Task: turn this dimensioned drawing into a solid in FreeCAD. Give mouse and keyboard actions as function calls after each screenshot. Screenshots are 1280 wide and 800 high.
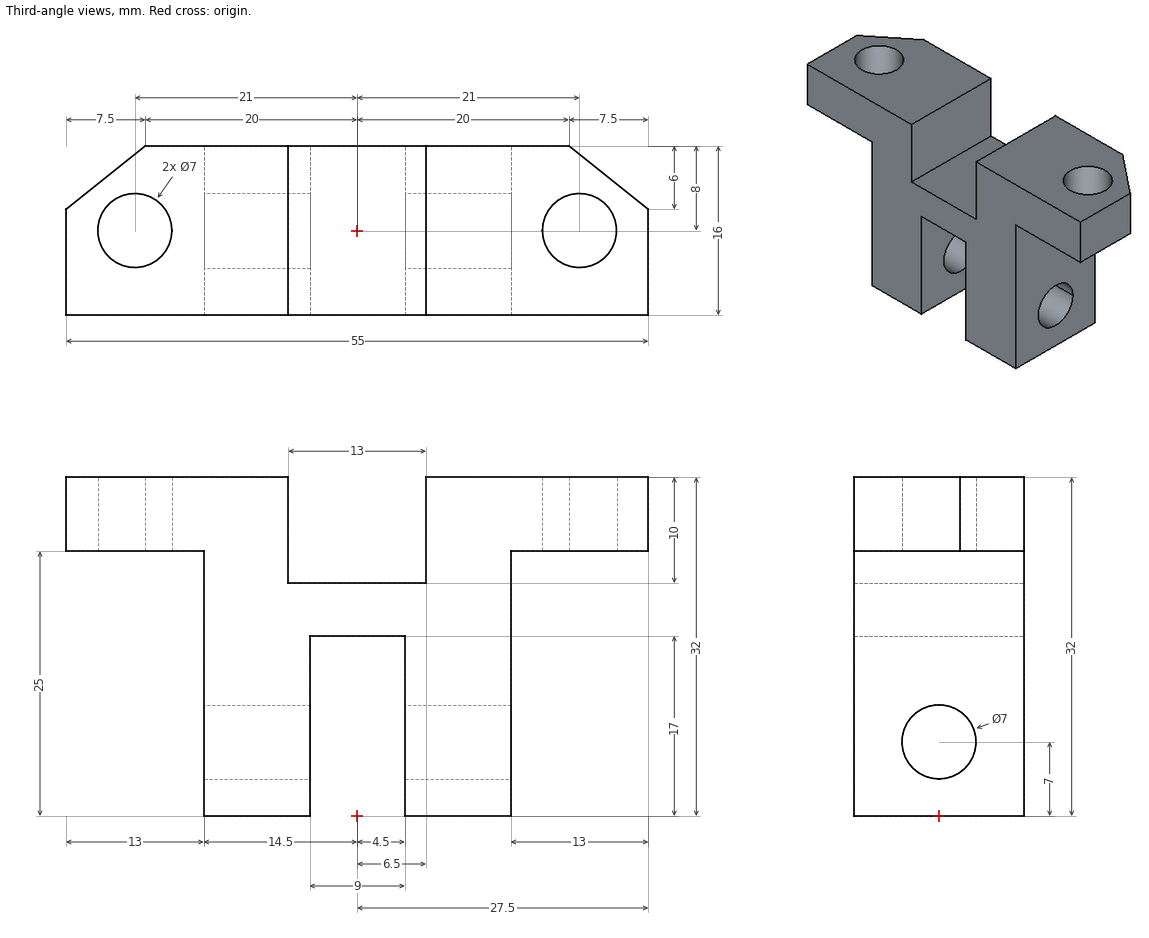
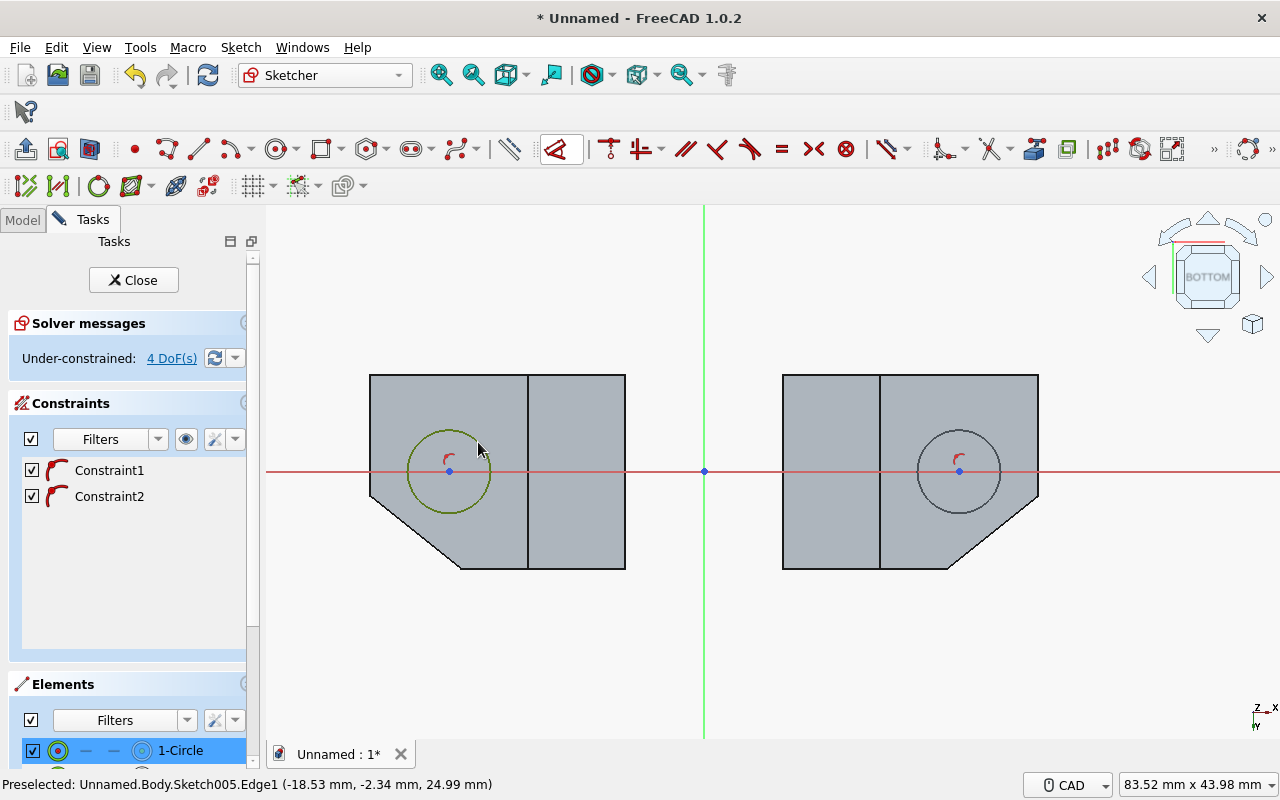
click(988, 442)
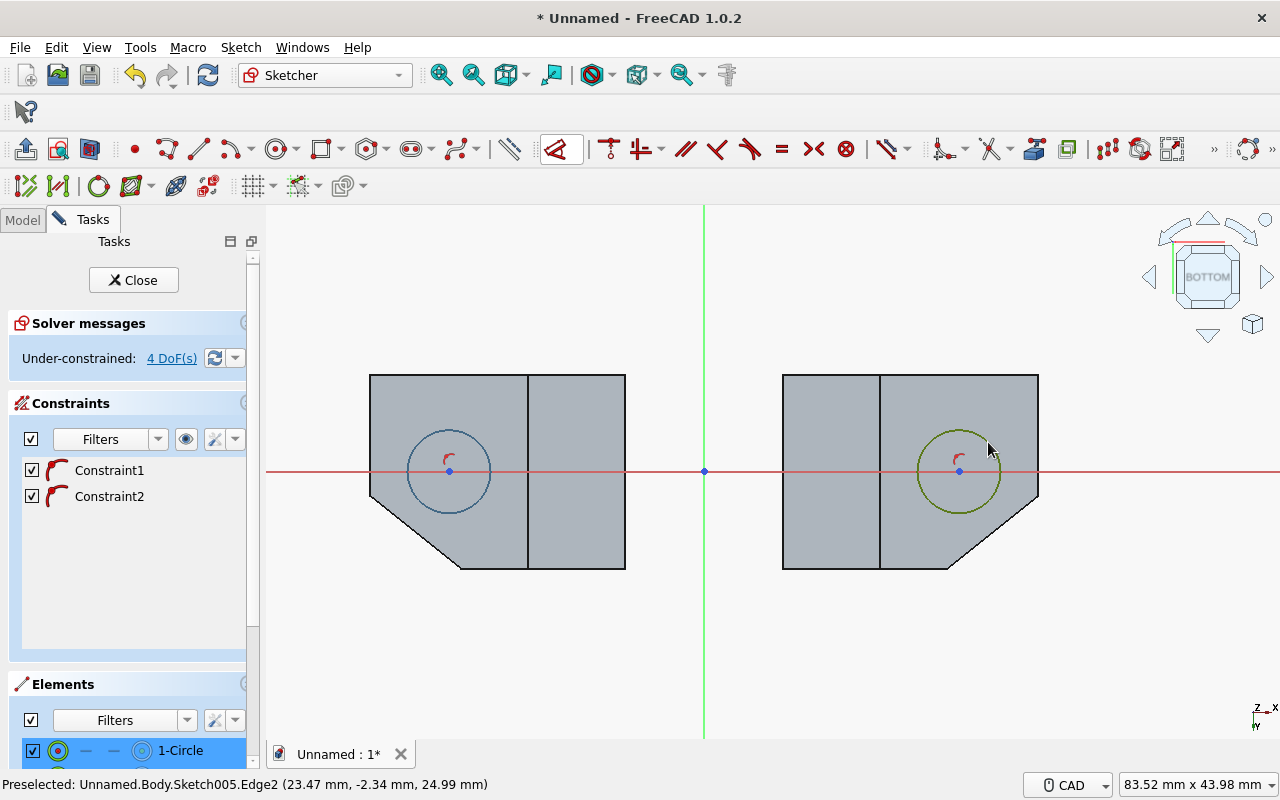
key(e)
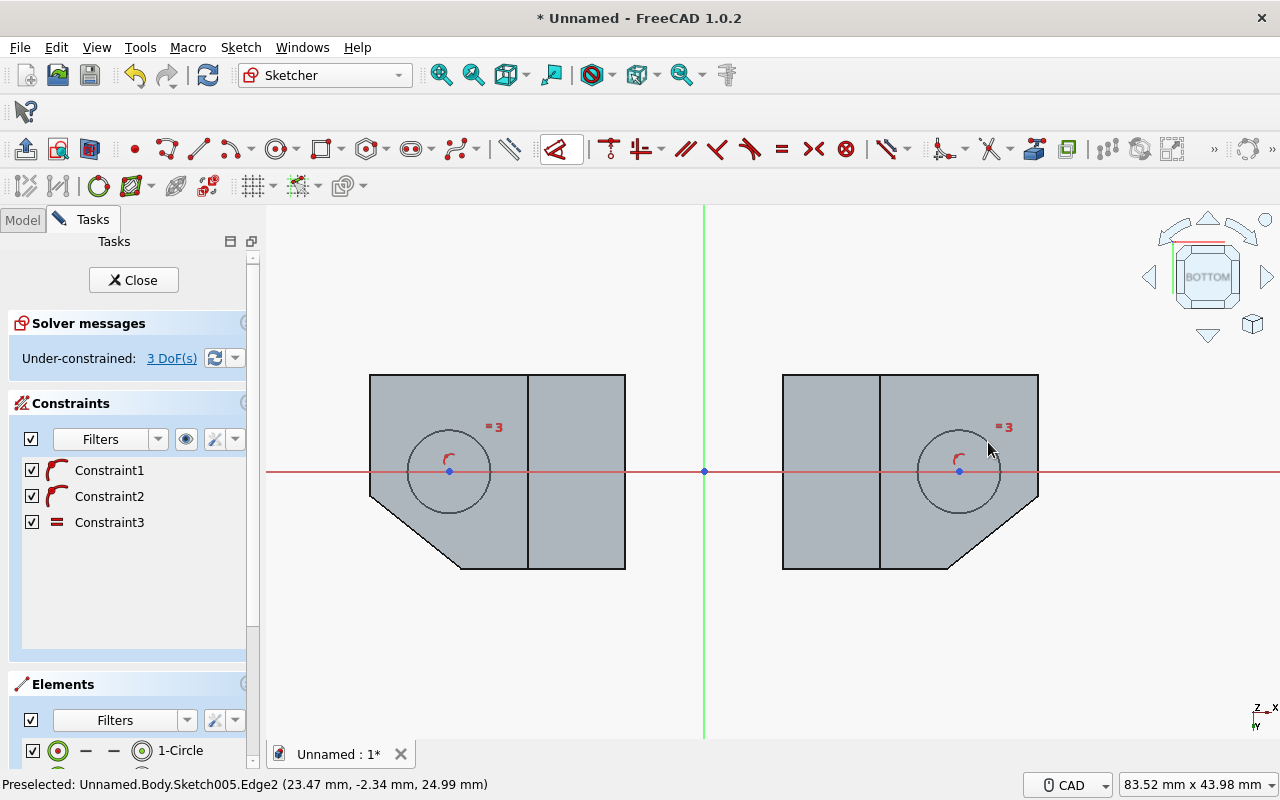
click(478, 442)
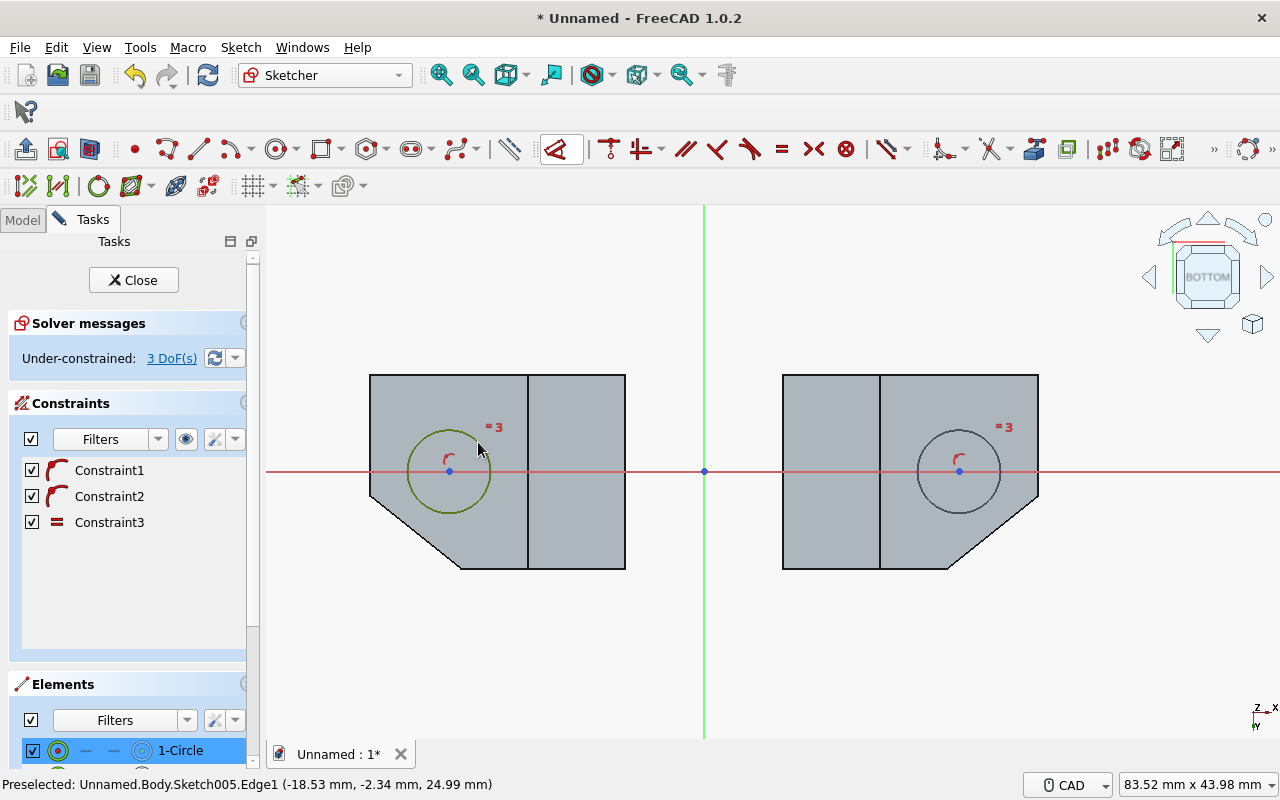
key(k)
key(o)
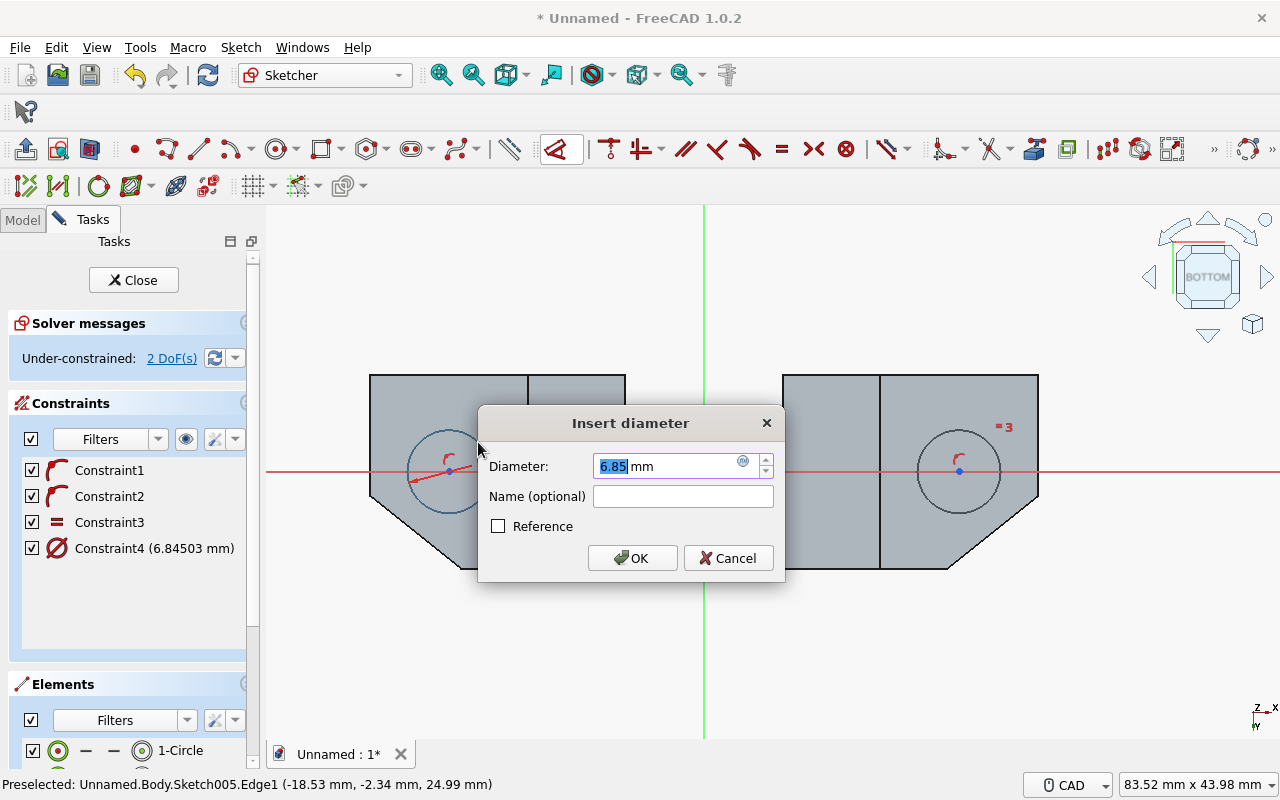
text(7)
key(Return)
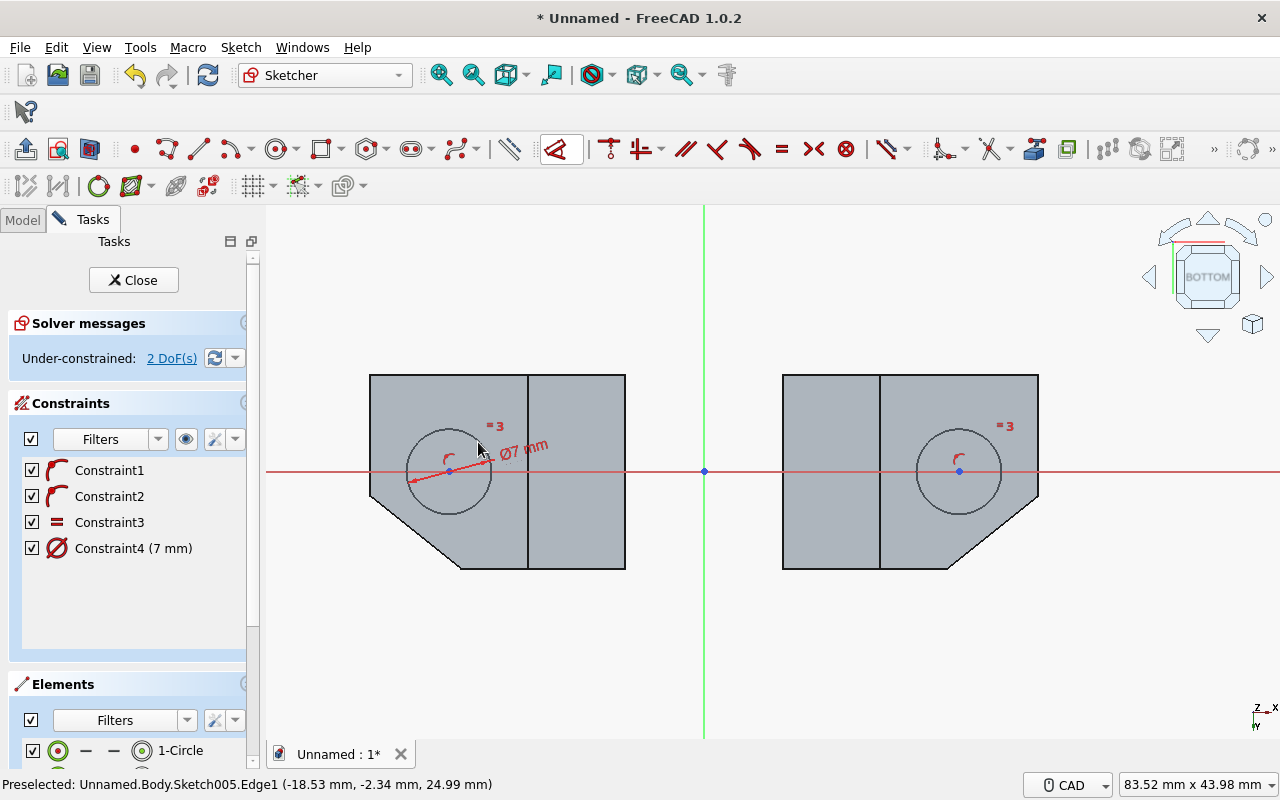
click(449, 472)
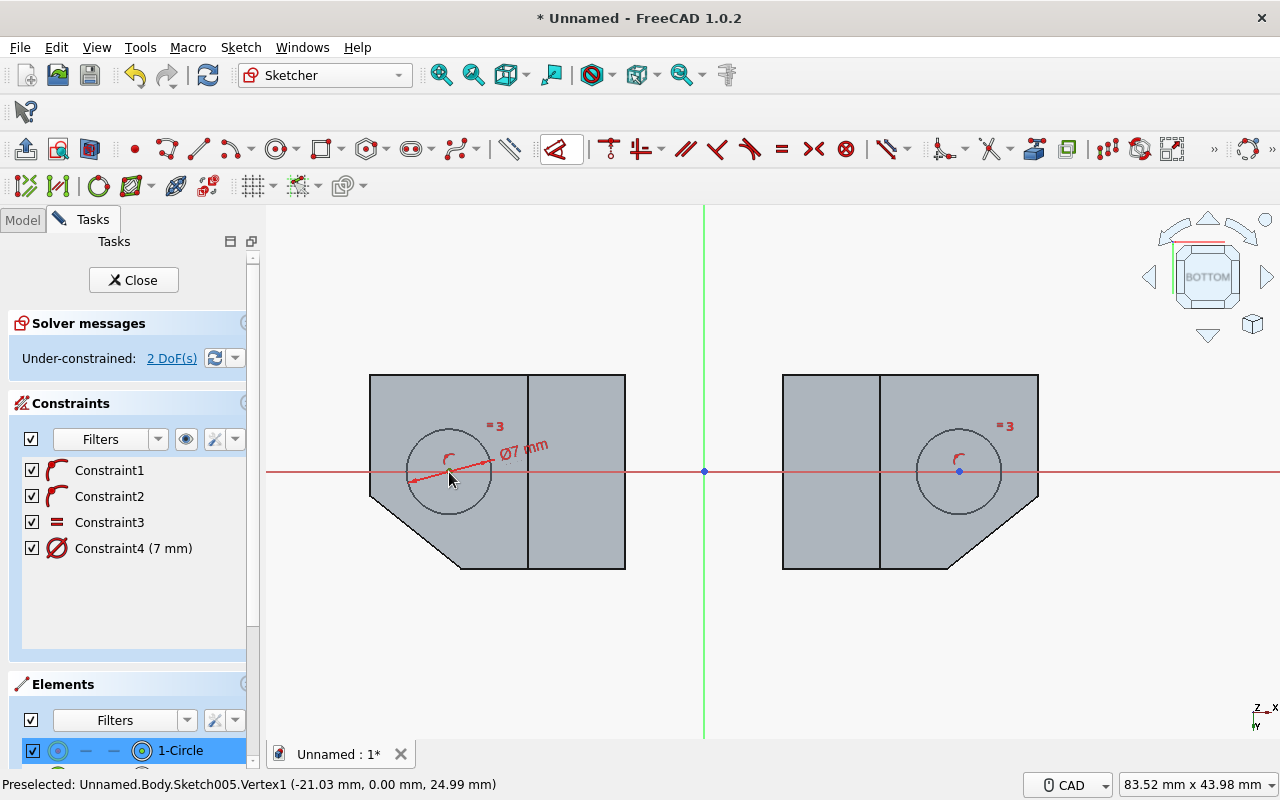
click(578, 150)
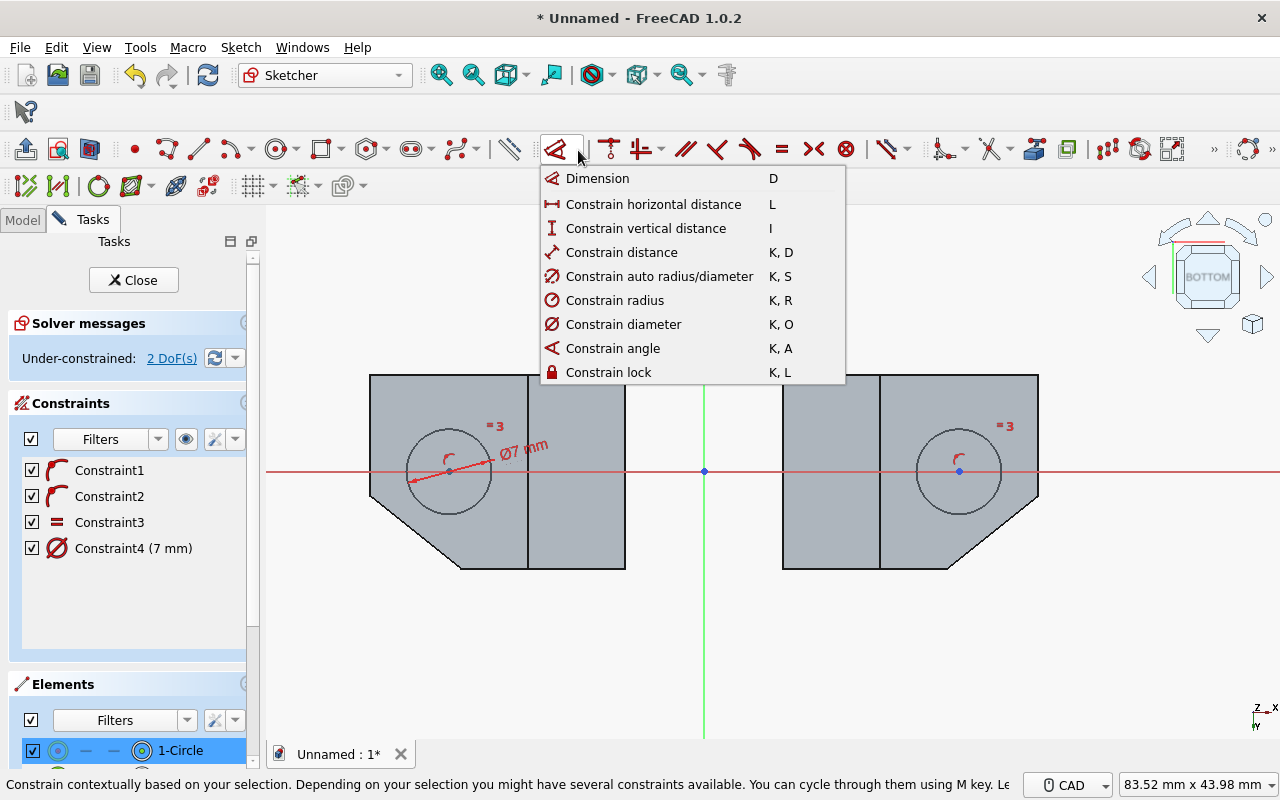
click(693, 204)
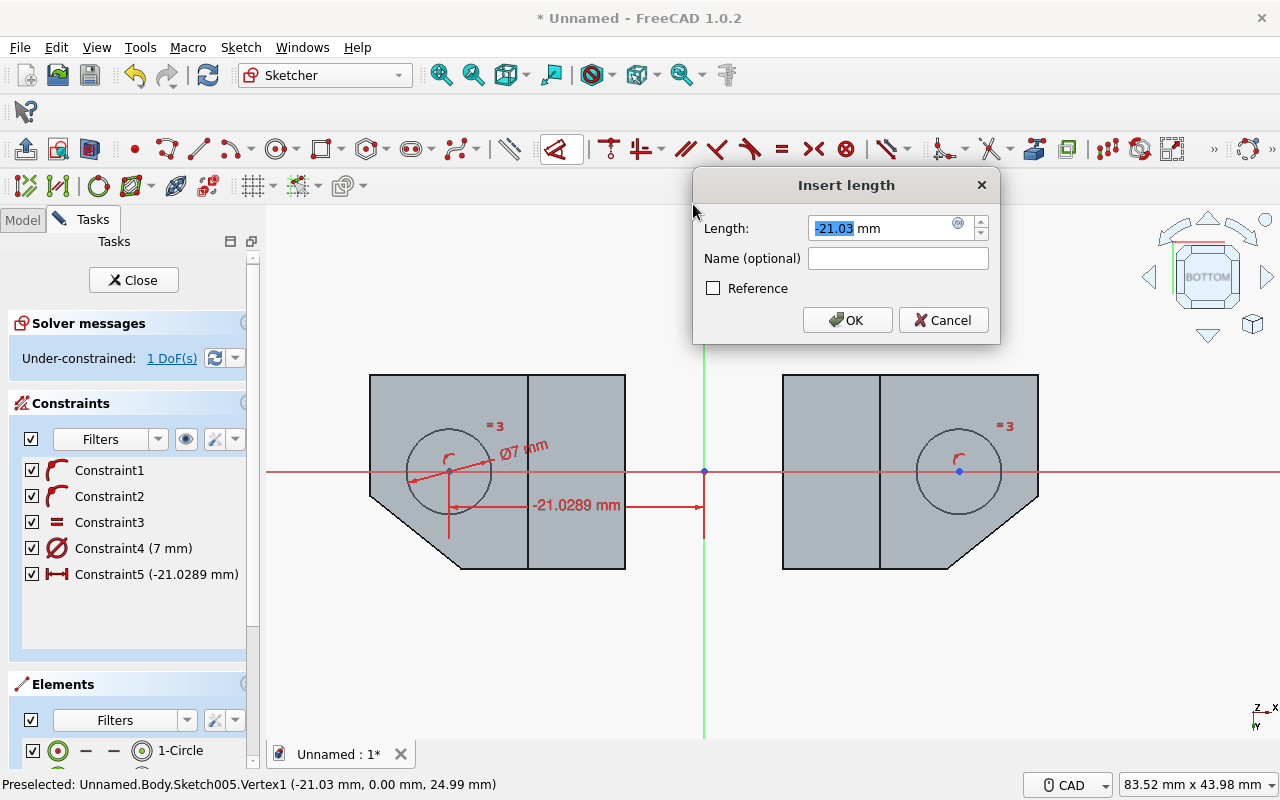
text(-21)
key(Return)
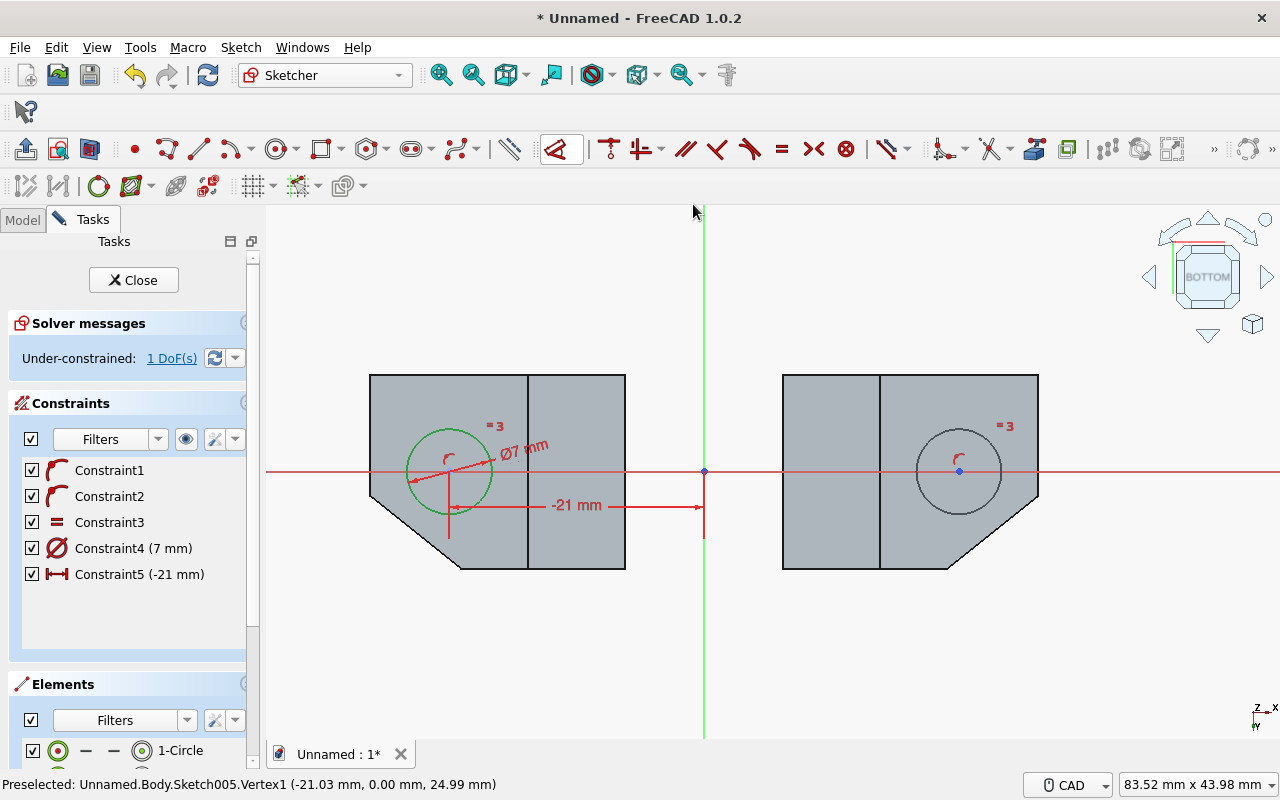
click(959, 472)